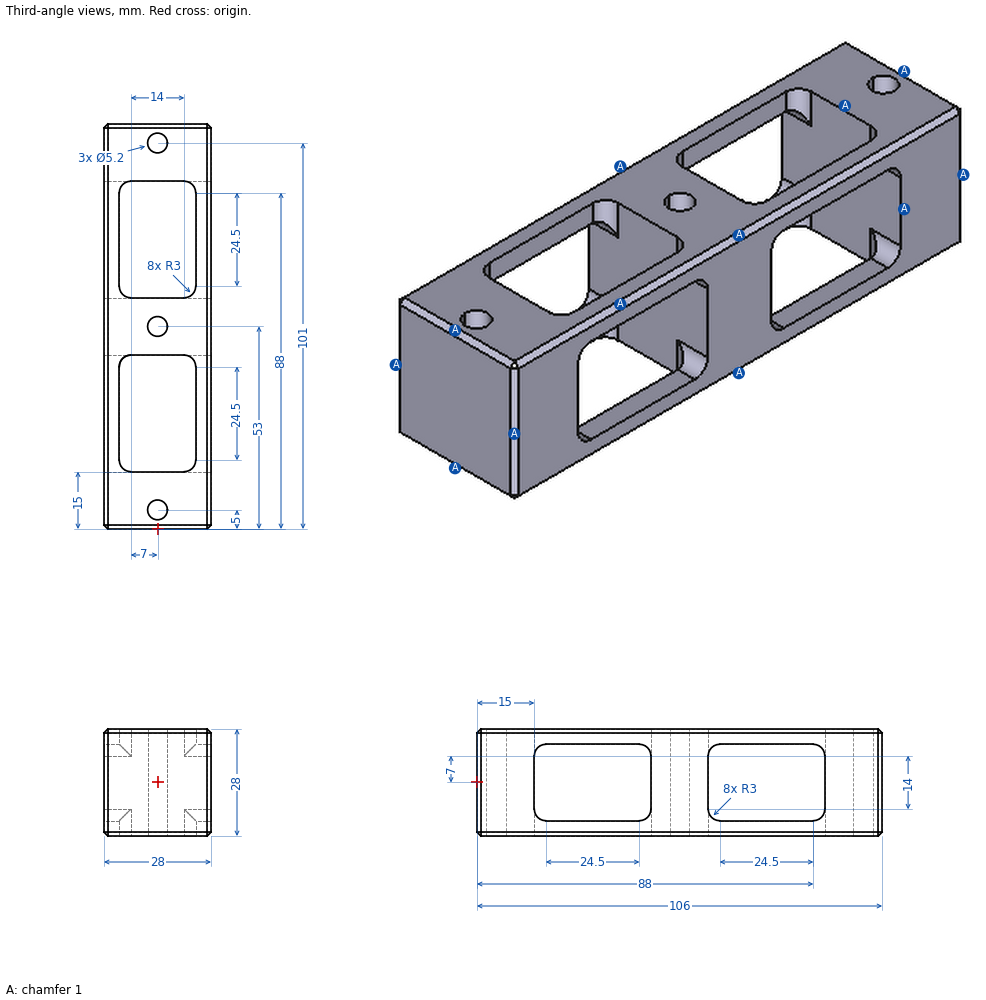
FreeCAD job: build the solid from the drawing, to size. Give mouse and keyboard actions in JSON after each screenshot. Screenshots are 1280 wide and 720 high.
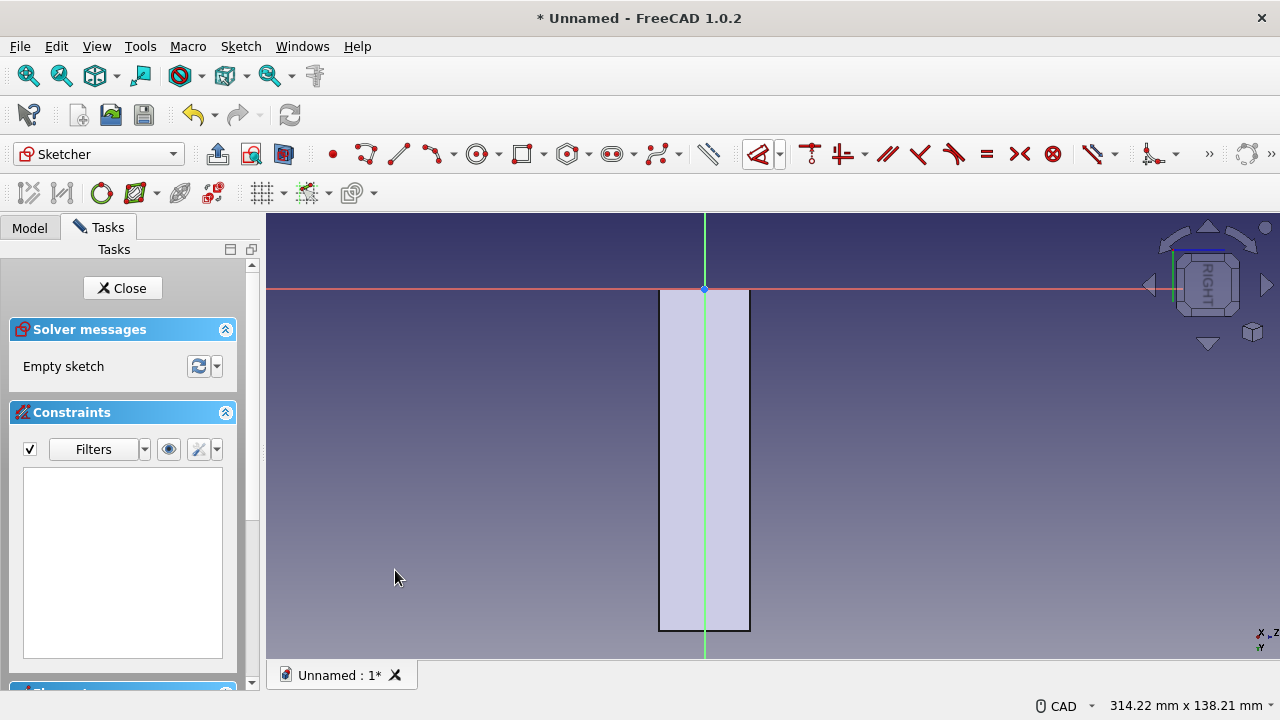
{"action": "left_click", "coordinate": [399, 154]}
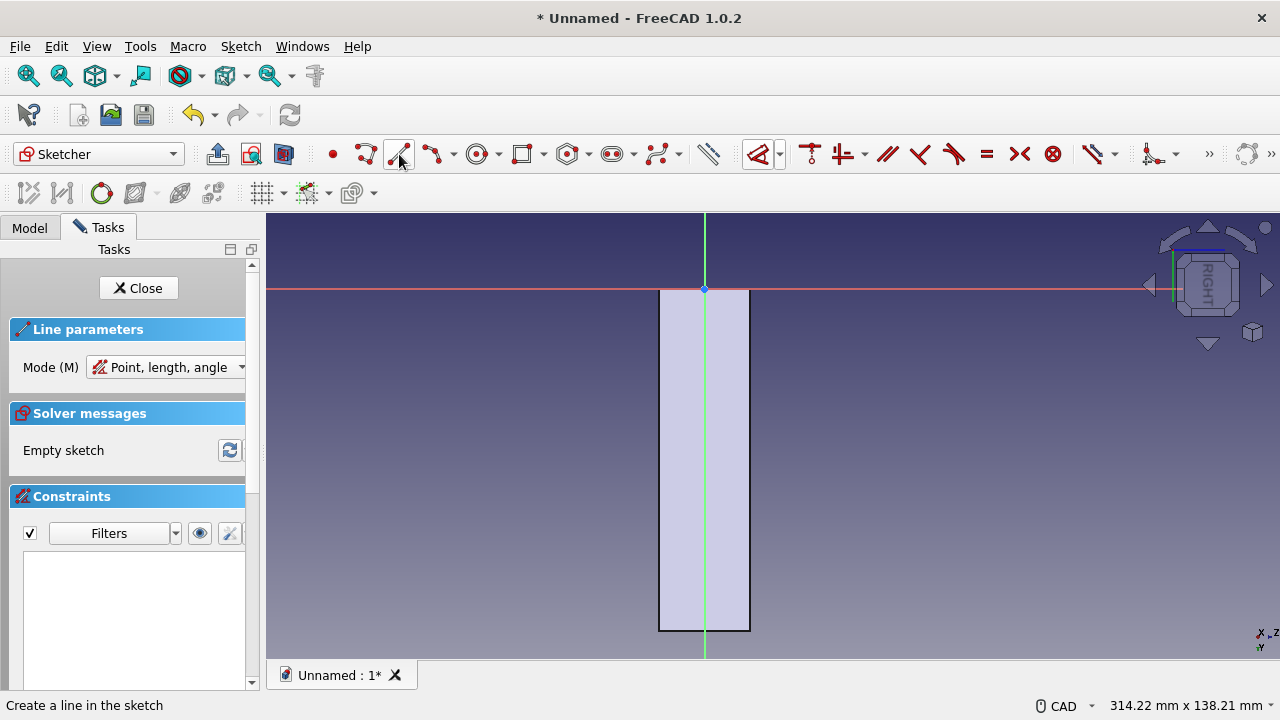
{"action": "left_click", "coordinate": [727, 485]}
{"action": "left_click", "coordinate": [682, 485]}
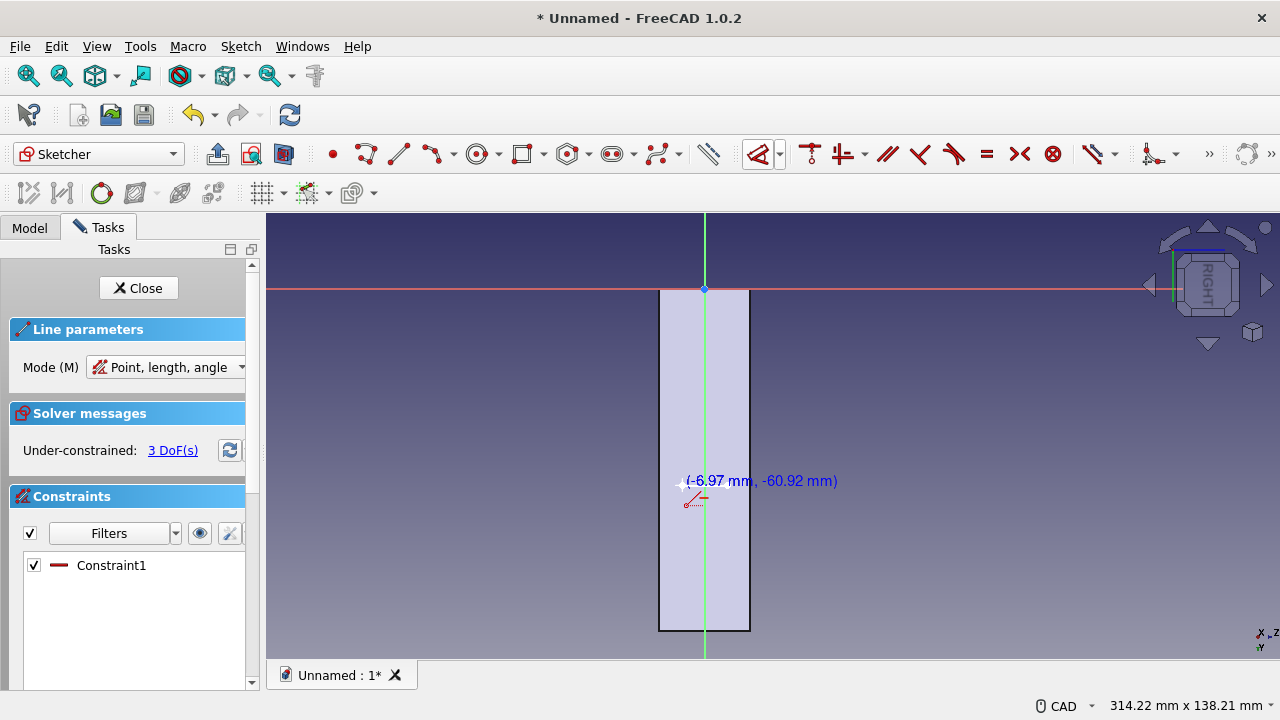
{"action": "left_click", "coordinate": [672, 494]}
{"action": "left_click", "coordinate": [672, 573]}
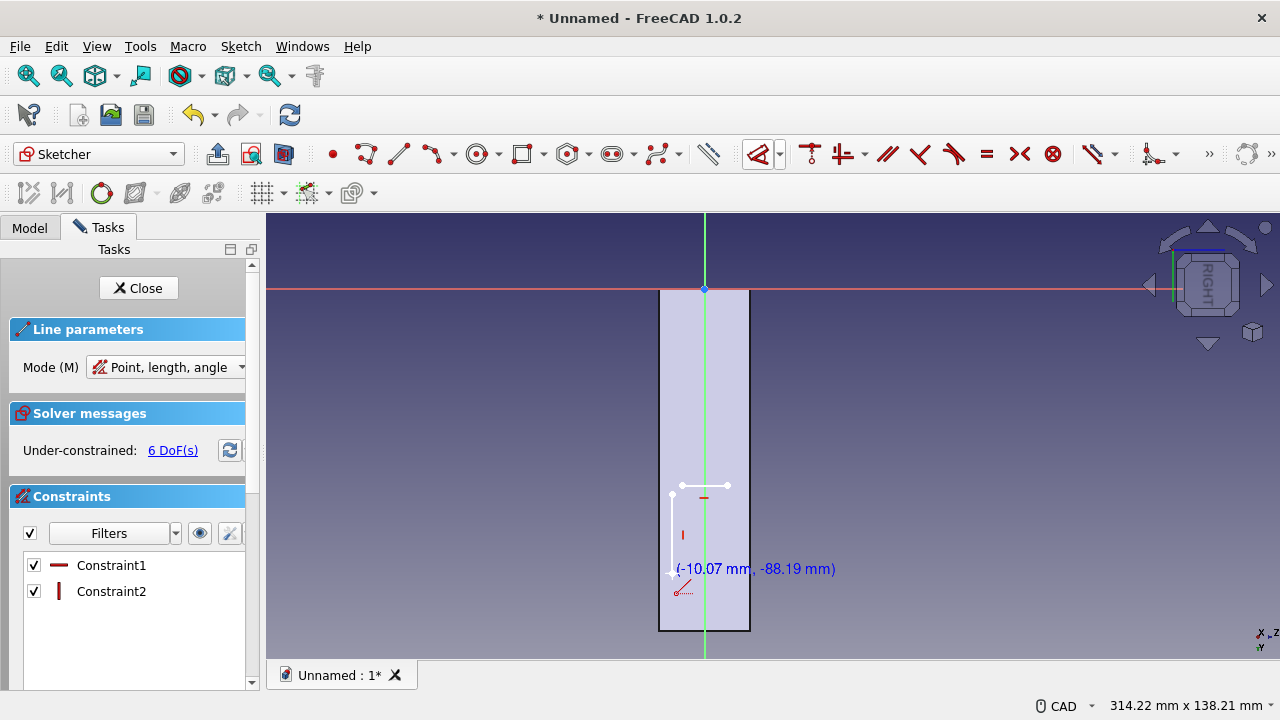
{"action": "left_click", "coordinate": [682, 583]}
{"action": "left_click", "coordinate": [727, 583]}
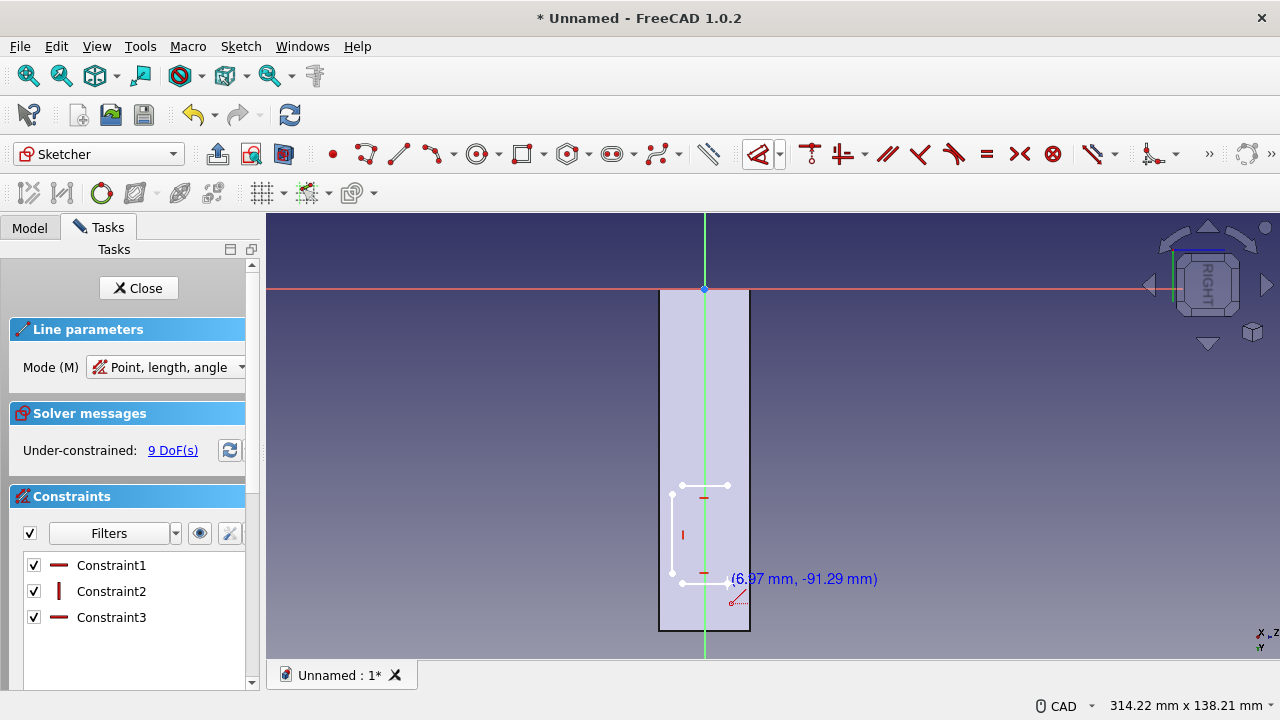
{"action": "left_click", "coordinate": [737, 573]}
{"action": "left_click", "coordinate": [737, 494]}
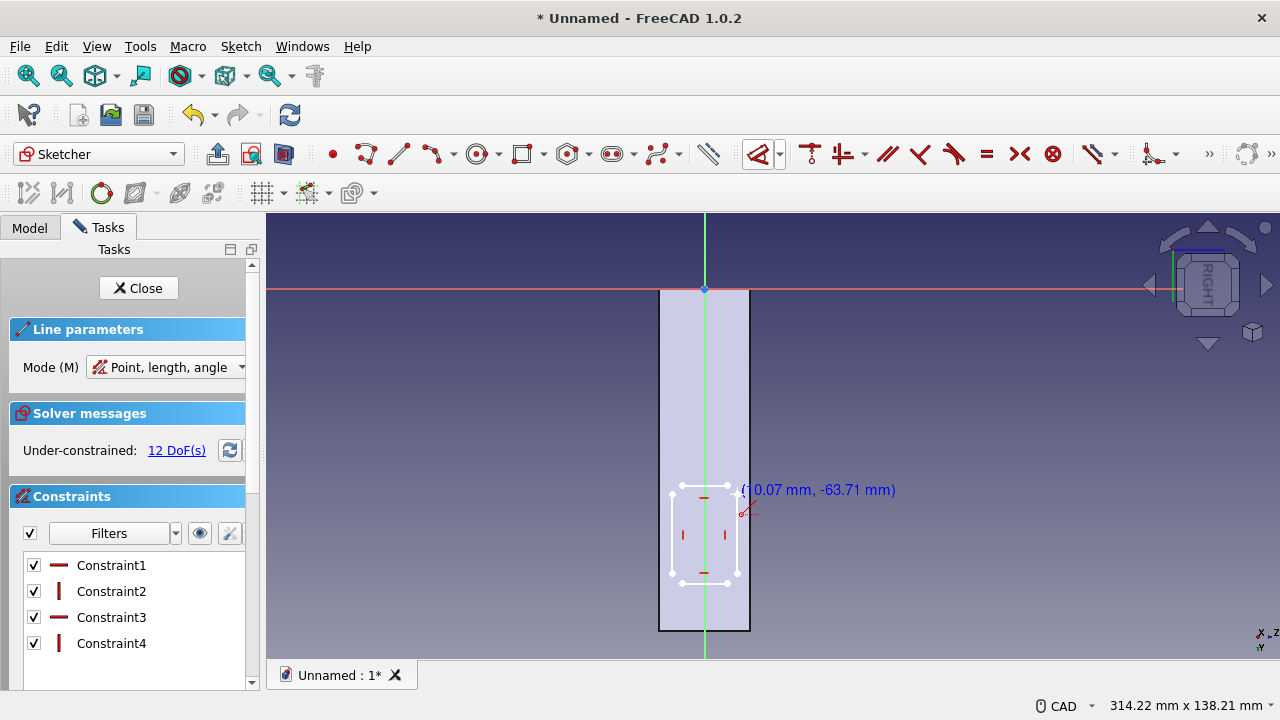
{"action": "left_click", "coordinate": [432, 154]}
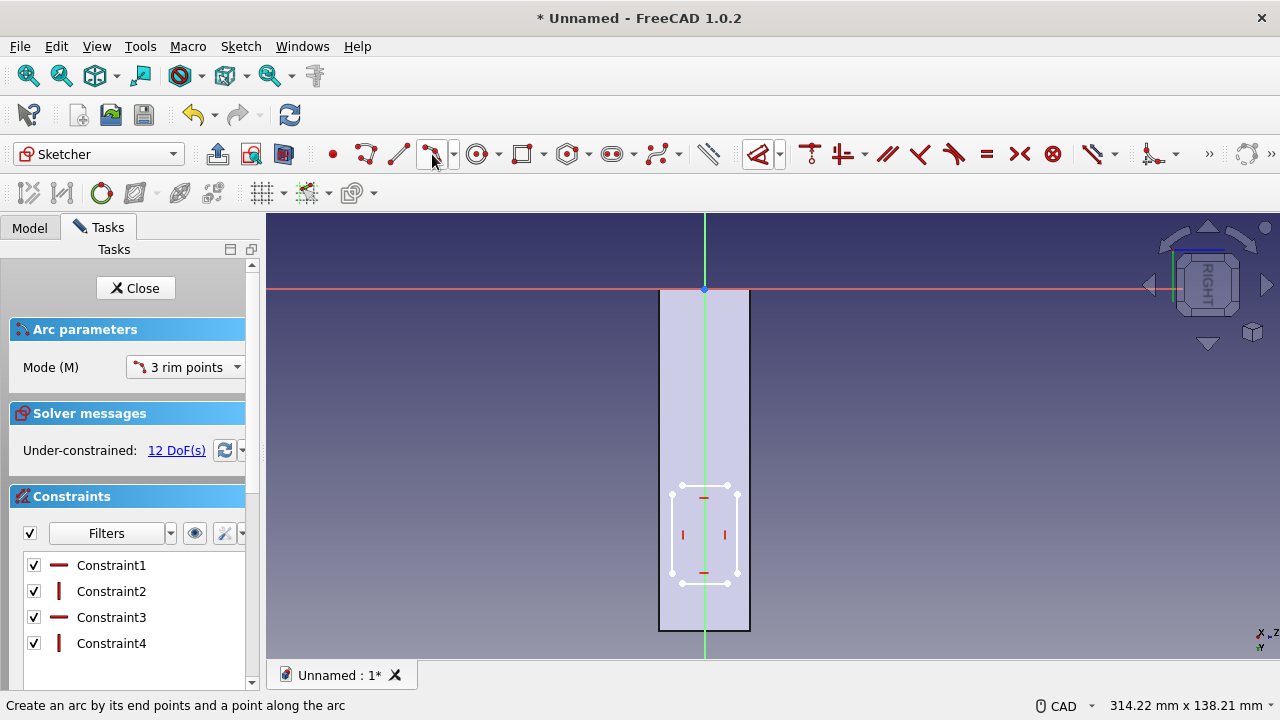
{"action": "left_click", "coordinate": [682, 486]}
{"action": "left_click", "coordinate": [672, 495]}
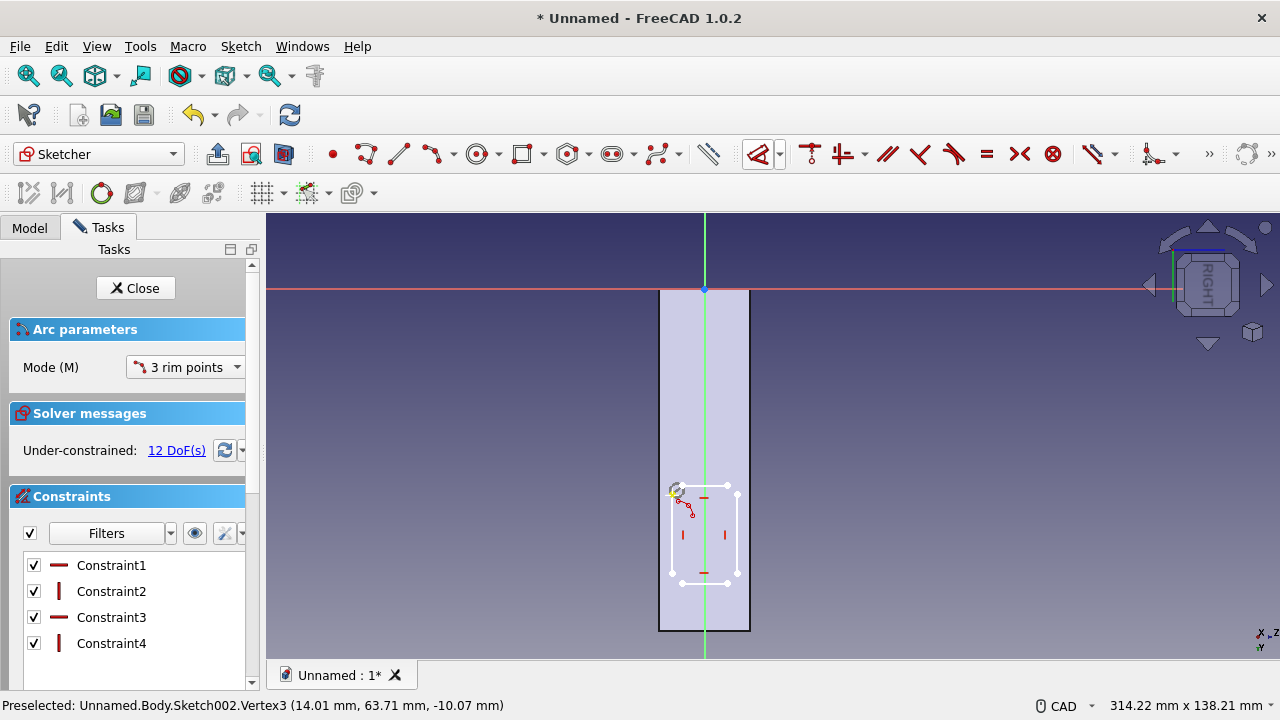
{"action": "scroll", "coordinate": [675, 487], "scroll_direction": "up", "scroll_amount": 9}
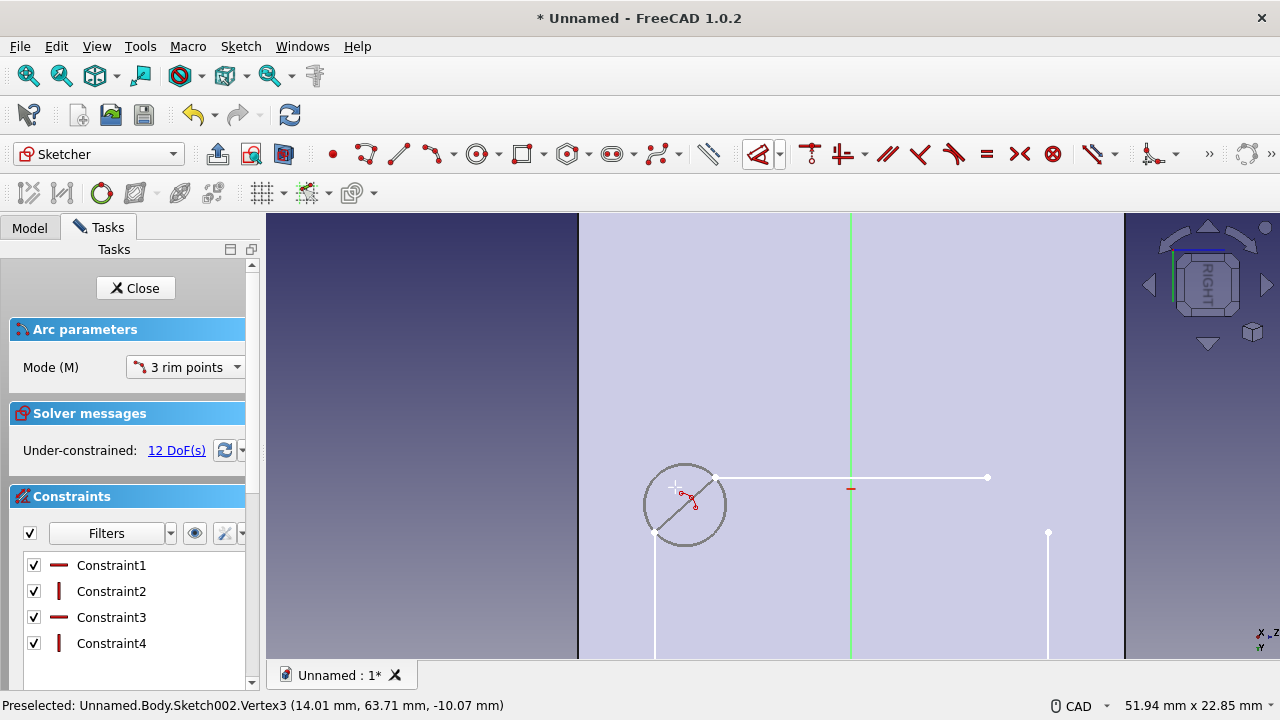
{"action": "left_click", "coordinate": [673, 487]}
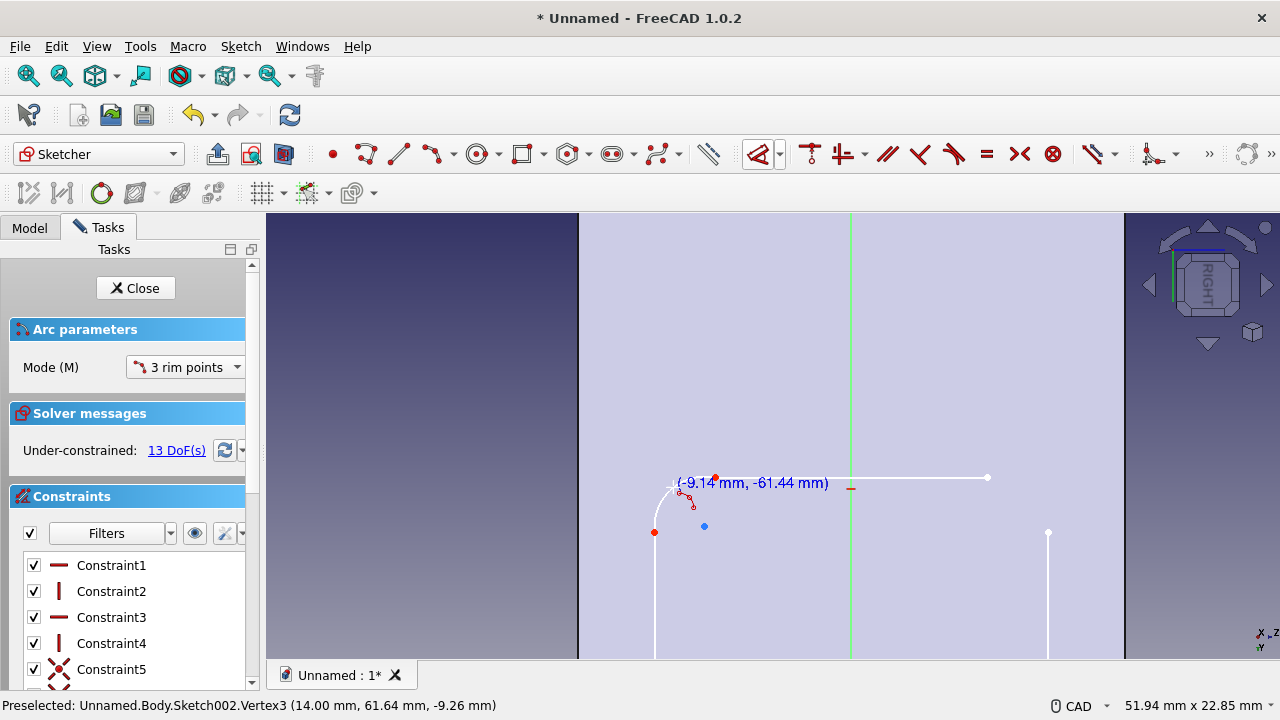
{"action": "scroll", "coordinate": [675, 487], "scroll_direction": "down", "scroll_amount": 9}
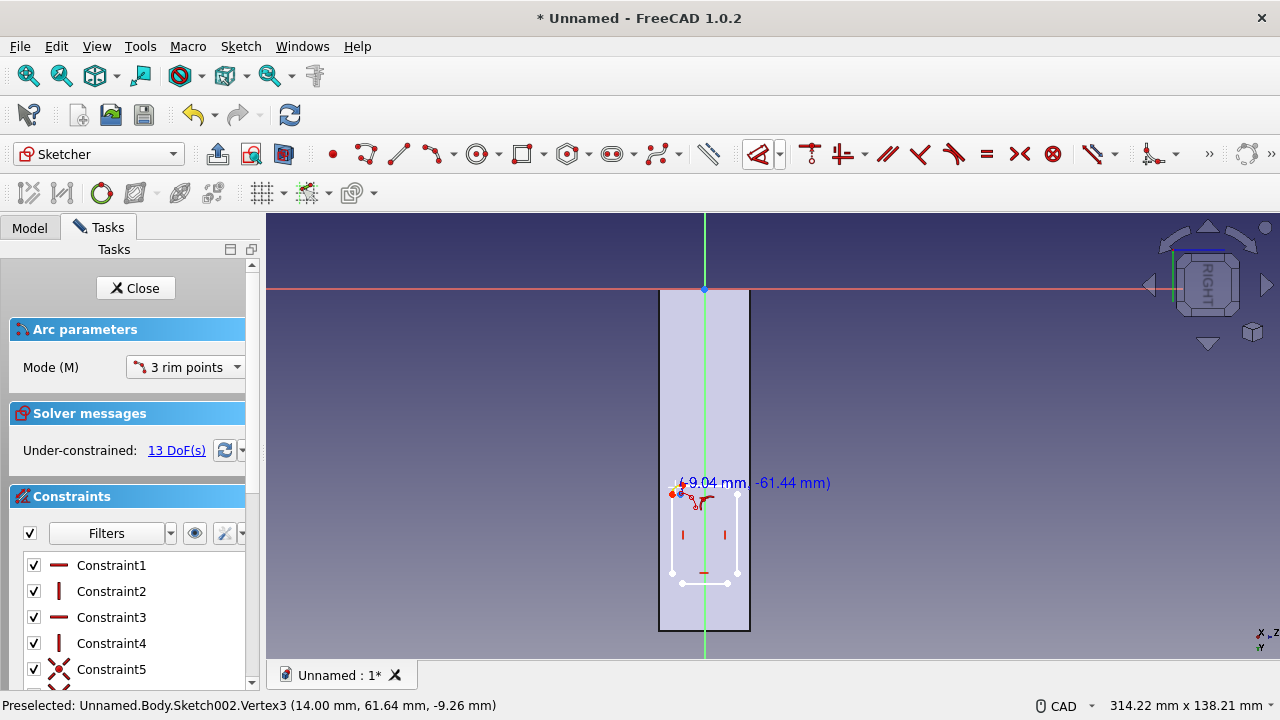
{"action": "left_click", "coordinate": [672, 574]}
{"action": "left_click", "coordinate": [682, 584]}